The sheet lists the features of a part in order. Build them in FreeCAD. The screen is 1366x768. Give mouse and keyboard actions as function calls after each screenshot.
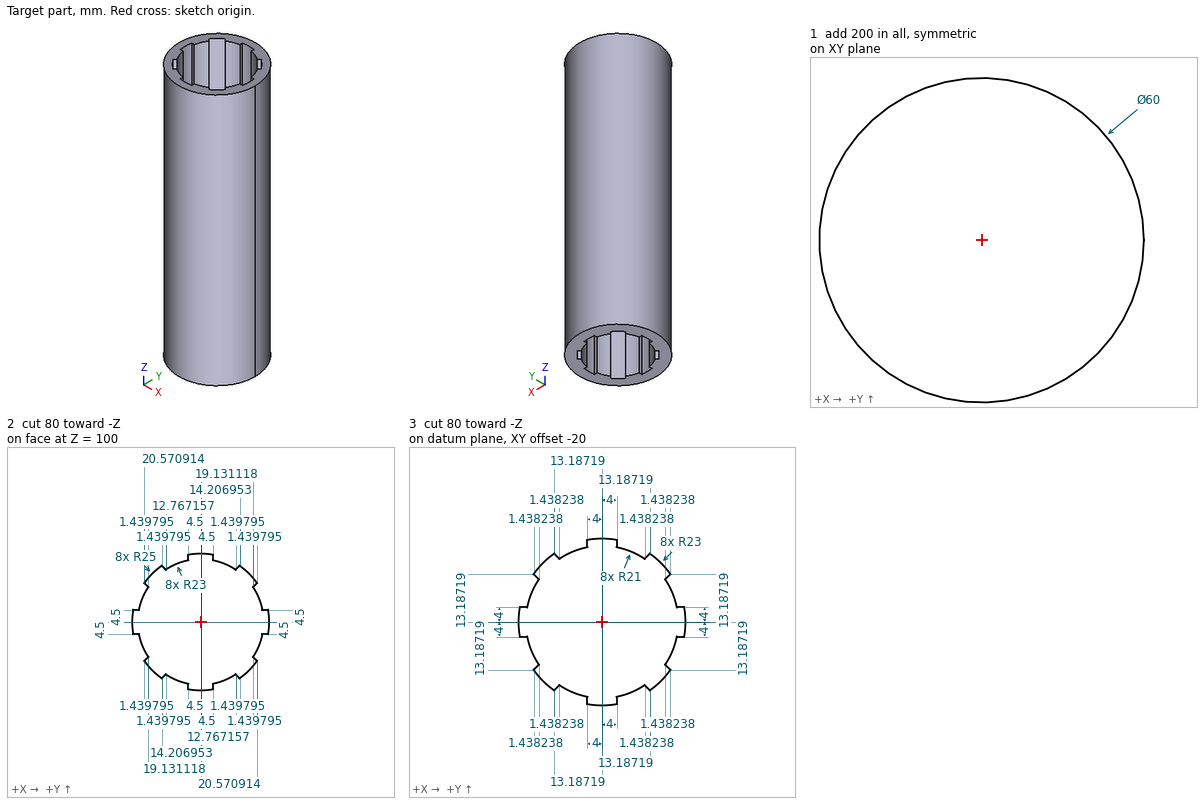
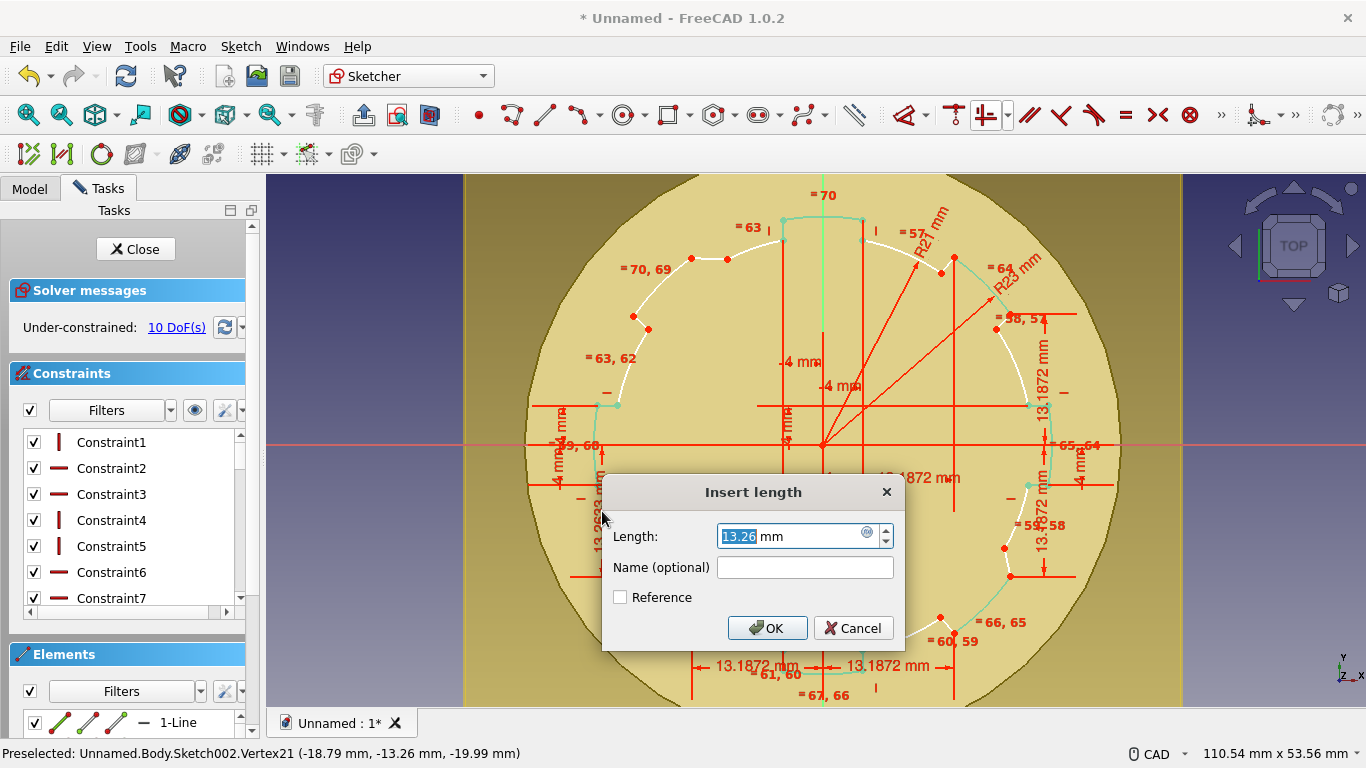
text(13.18719)
key(Return)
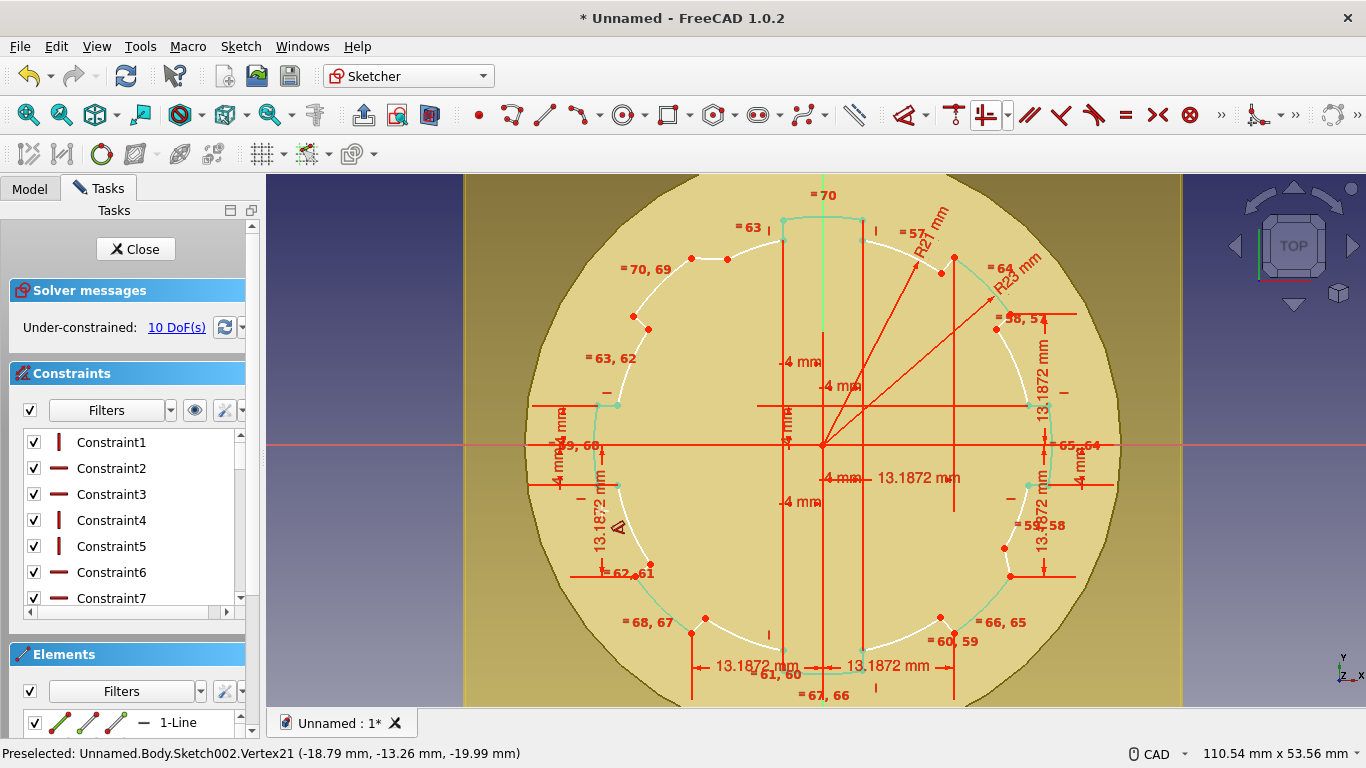
click(634, 316)
click(600, 381)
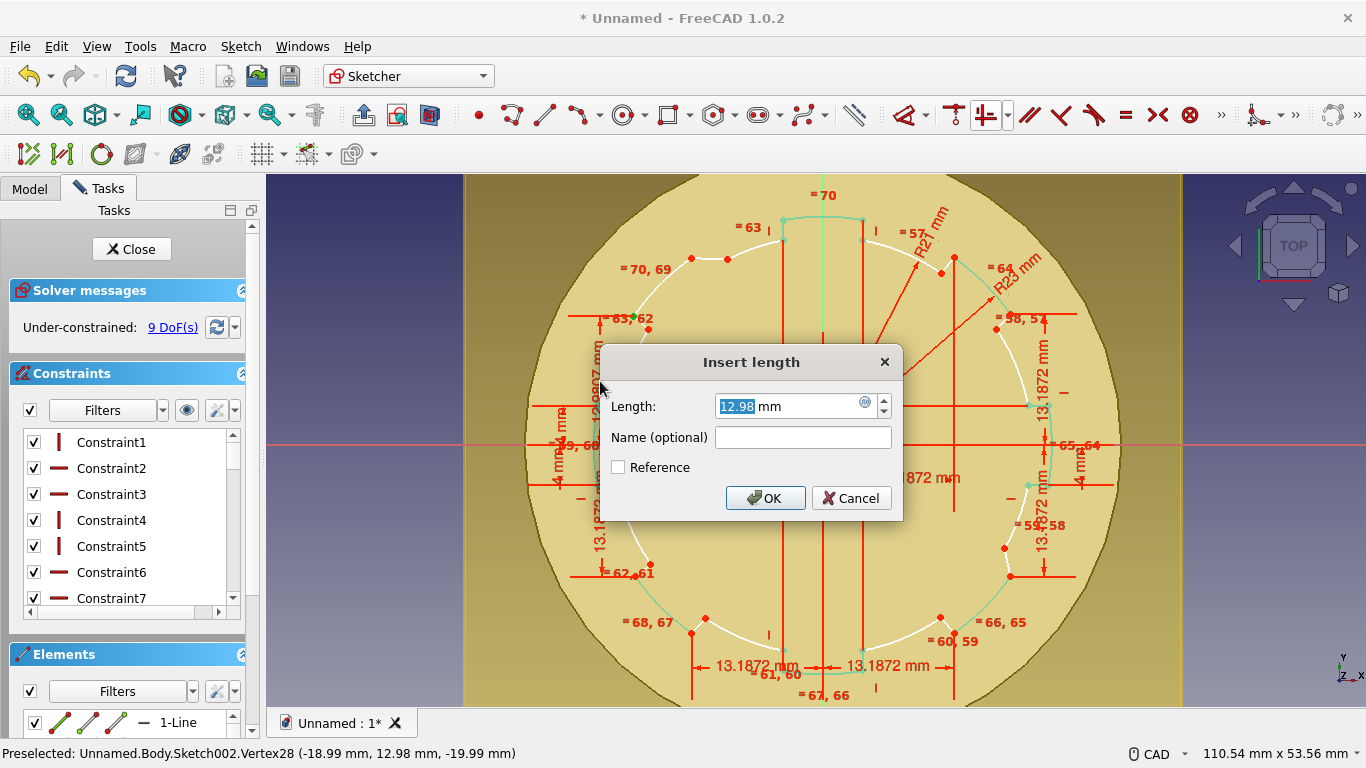
text(13.18719)
key(Return)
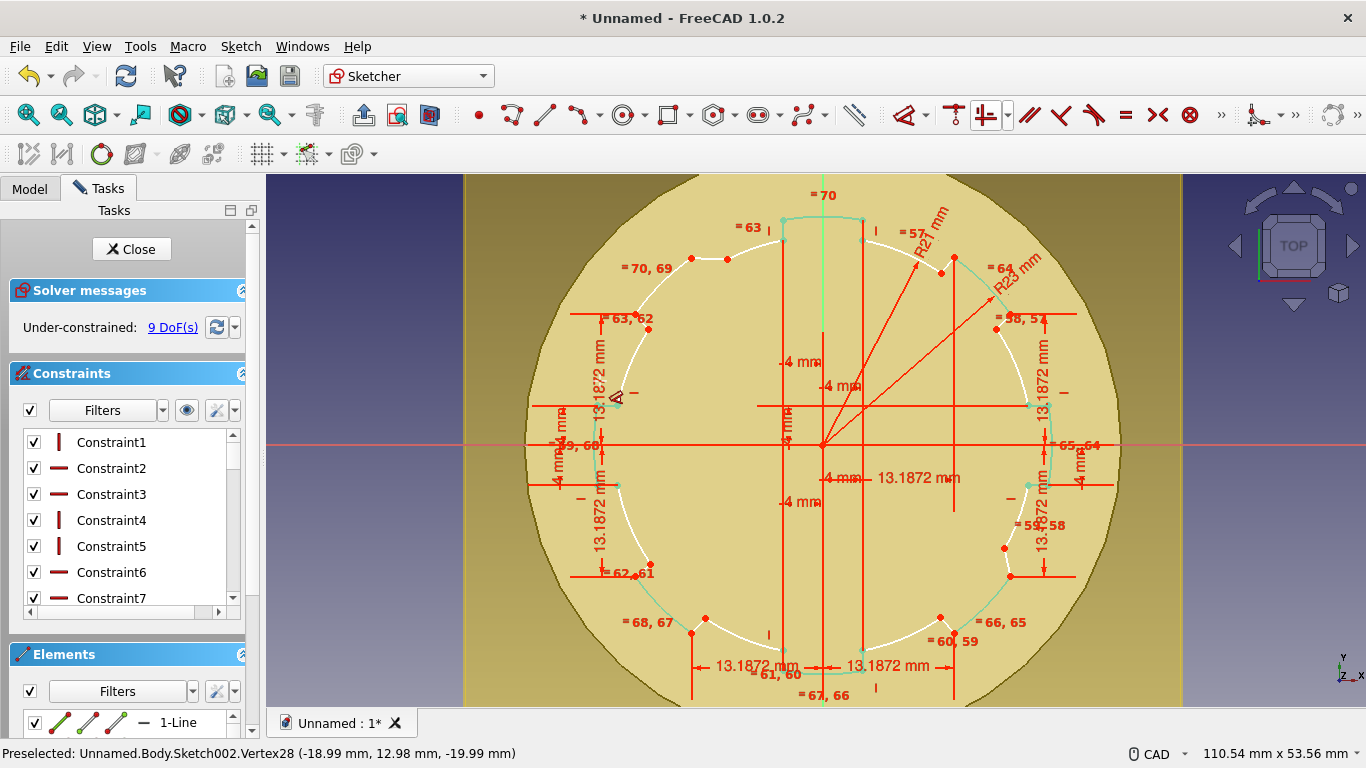
click(691, 258)
click(757, 224)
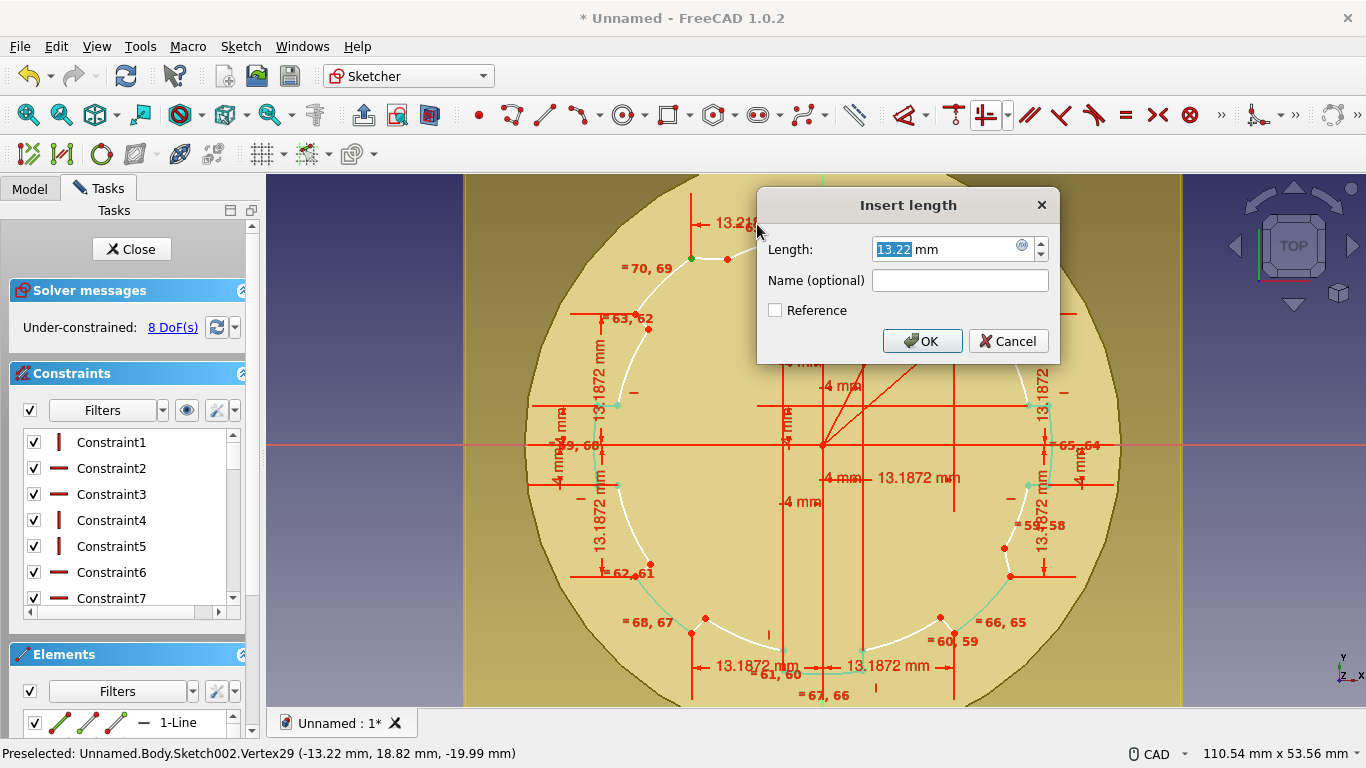
text(13.18719)
key(Return)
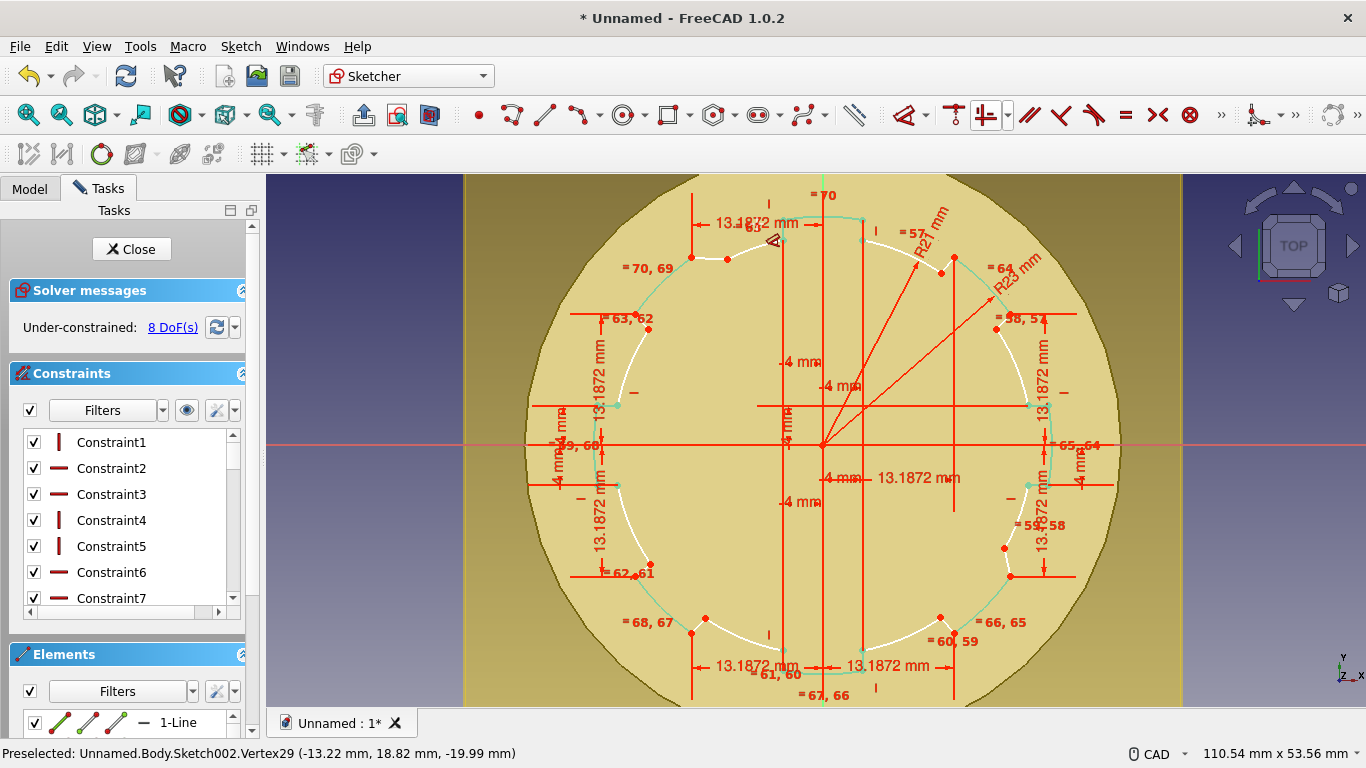
scroll(948, 266, up, 6)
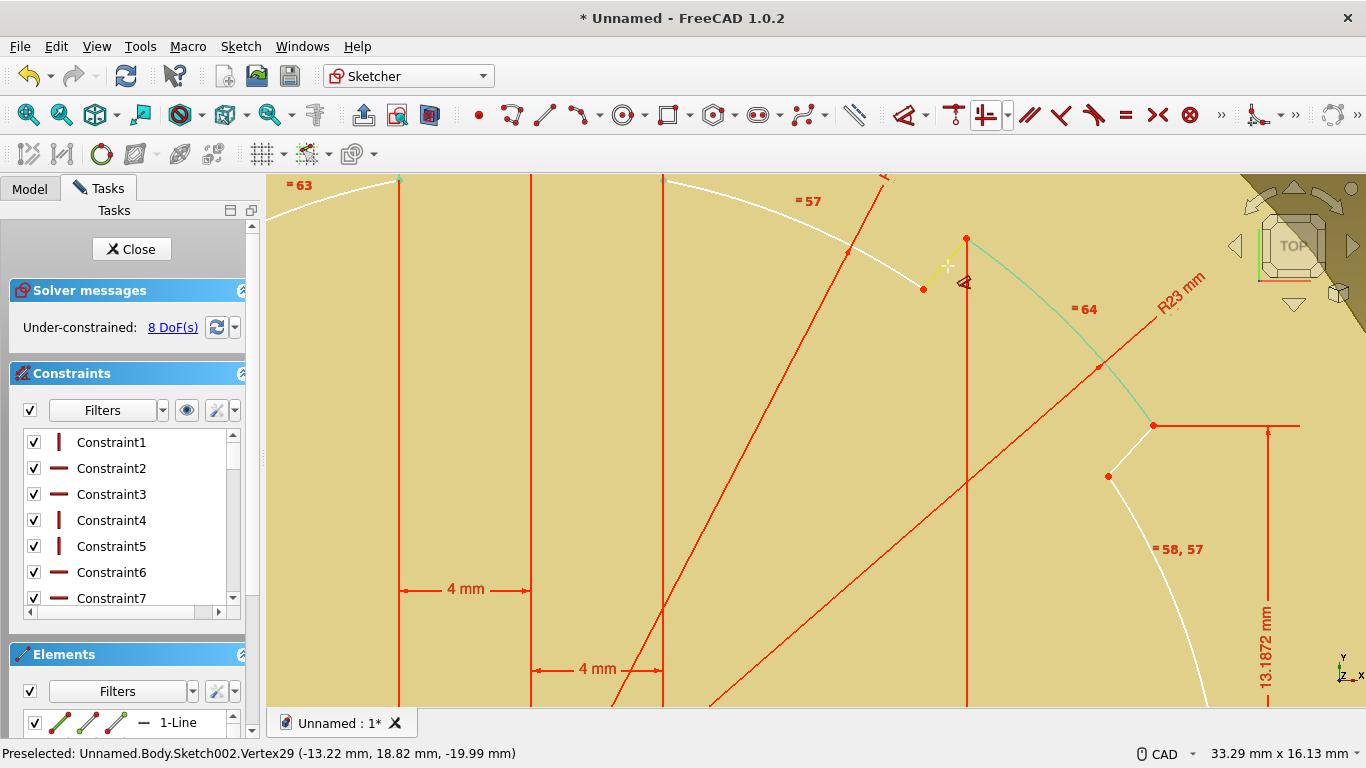
click(945, 264)
click(945, 205)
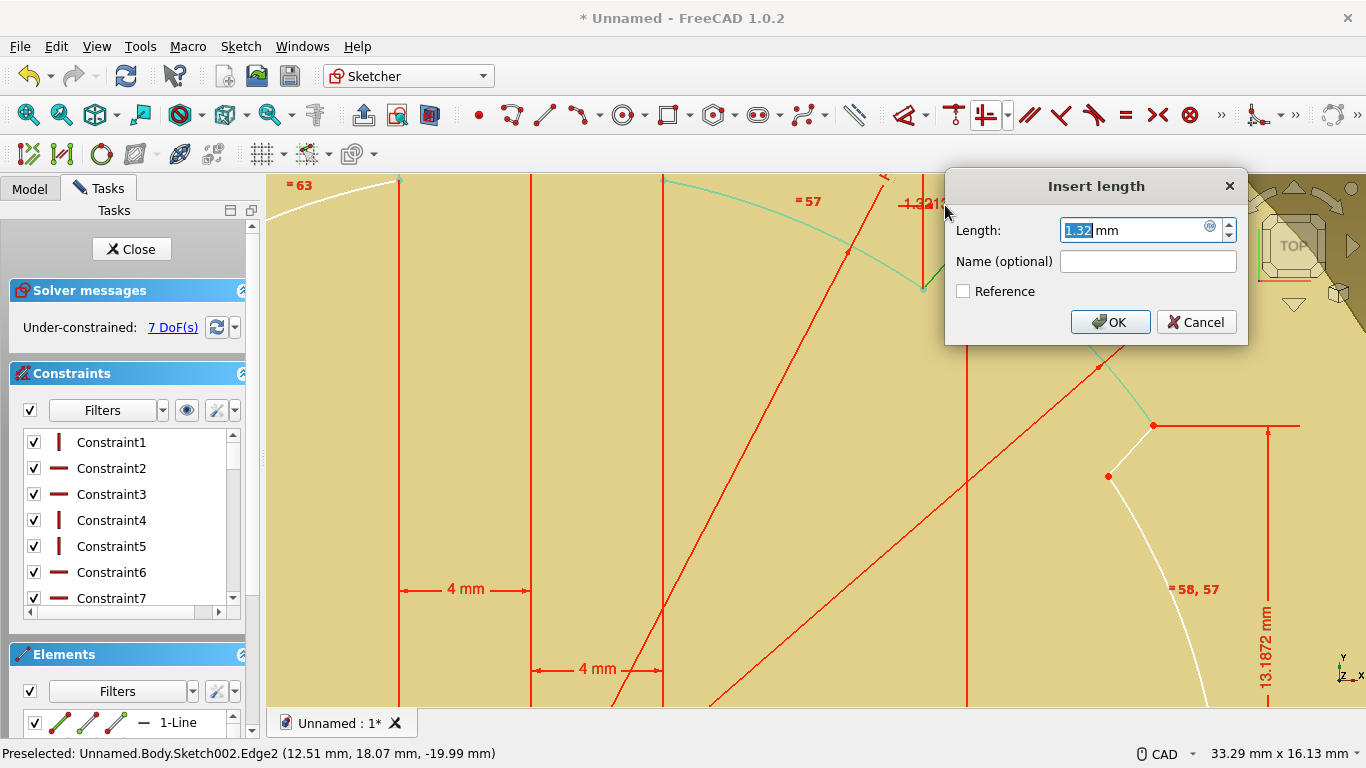
text(1.438238)
key(Return)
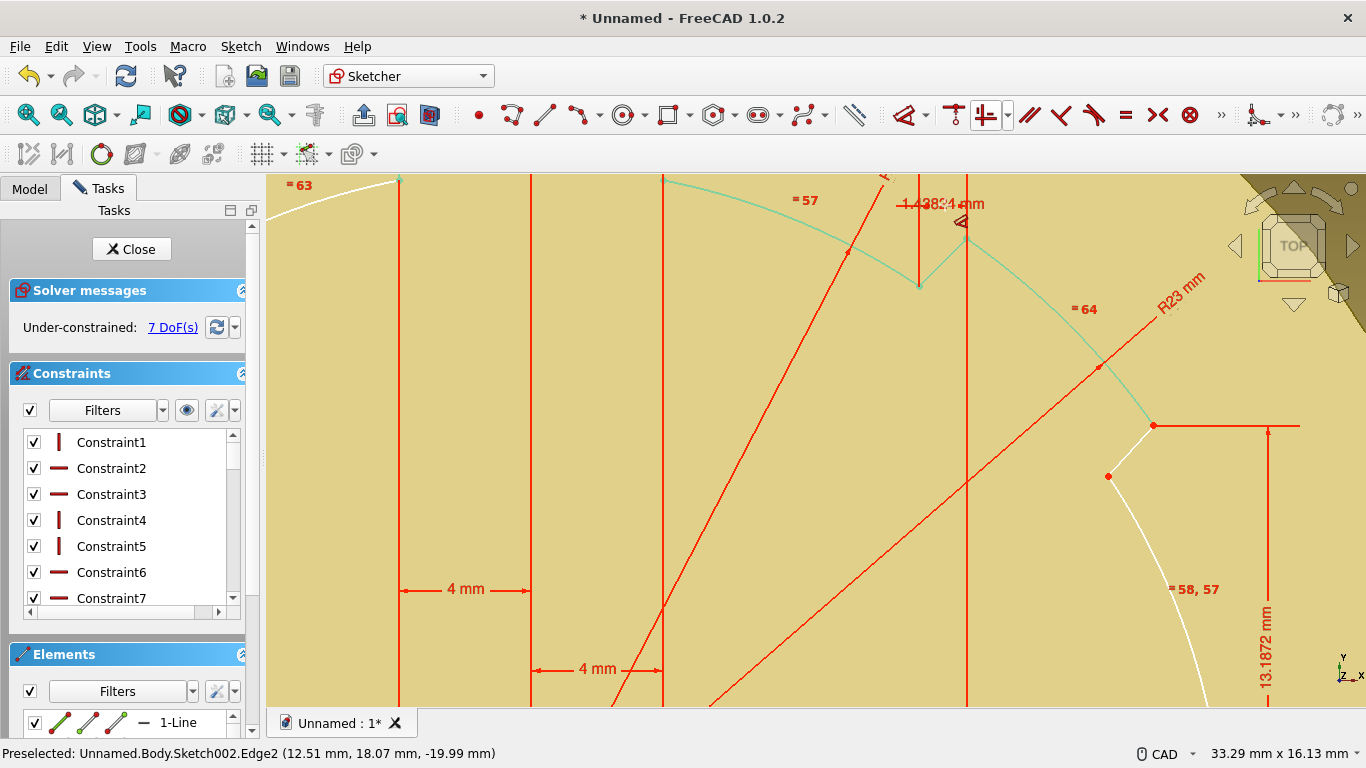
click(1140, 441)
click(1147, 392)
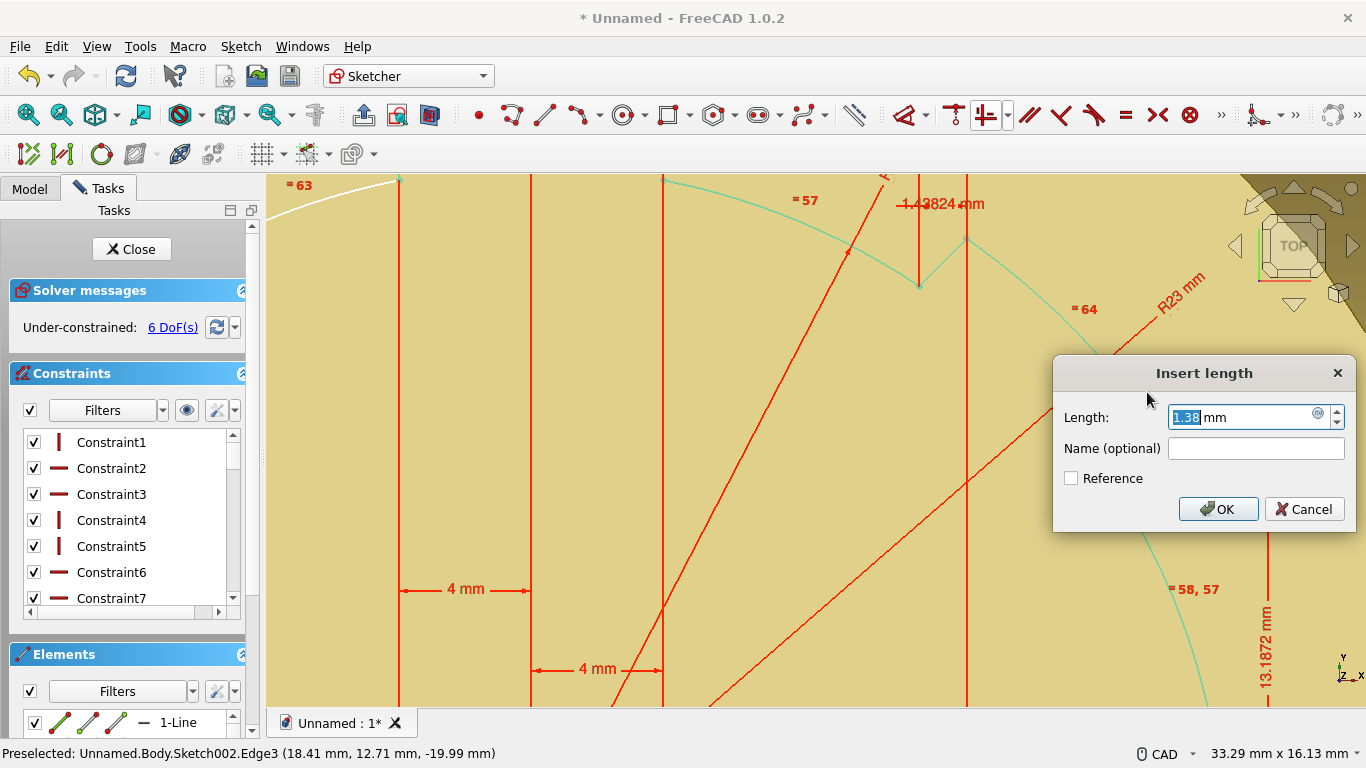
text(1.438238)
key(Return)